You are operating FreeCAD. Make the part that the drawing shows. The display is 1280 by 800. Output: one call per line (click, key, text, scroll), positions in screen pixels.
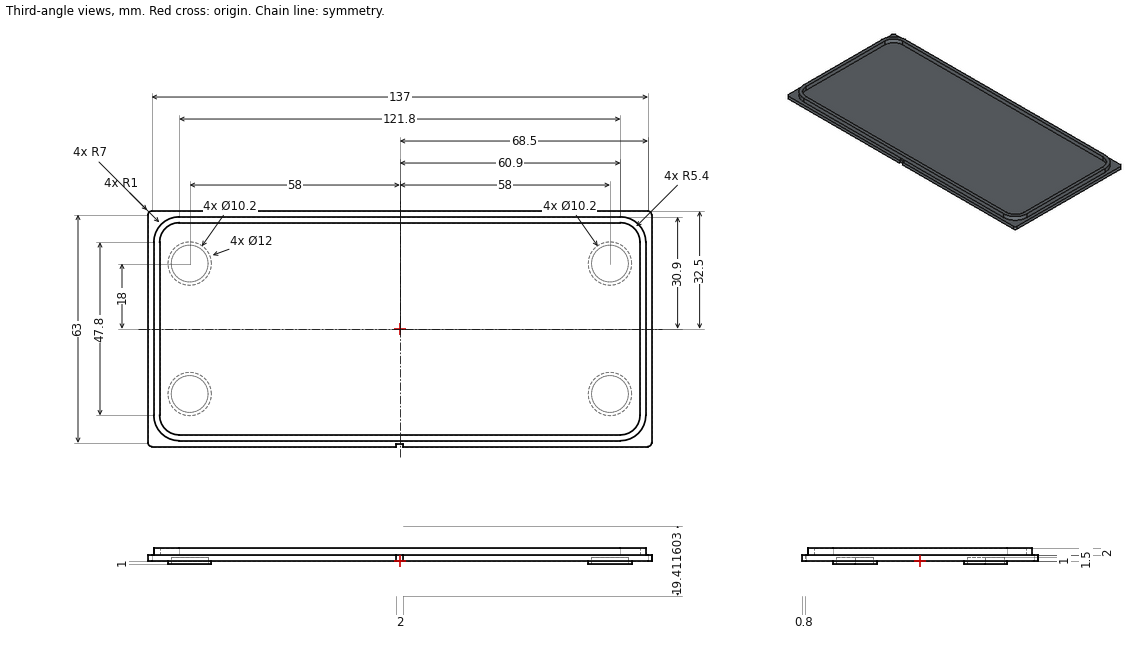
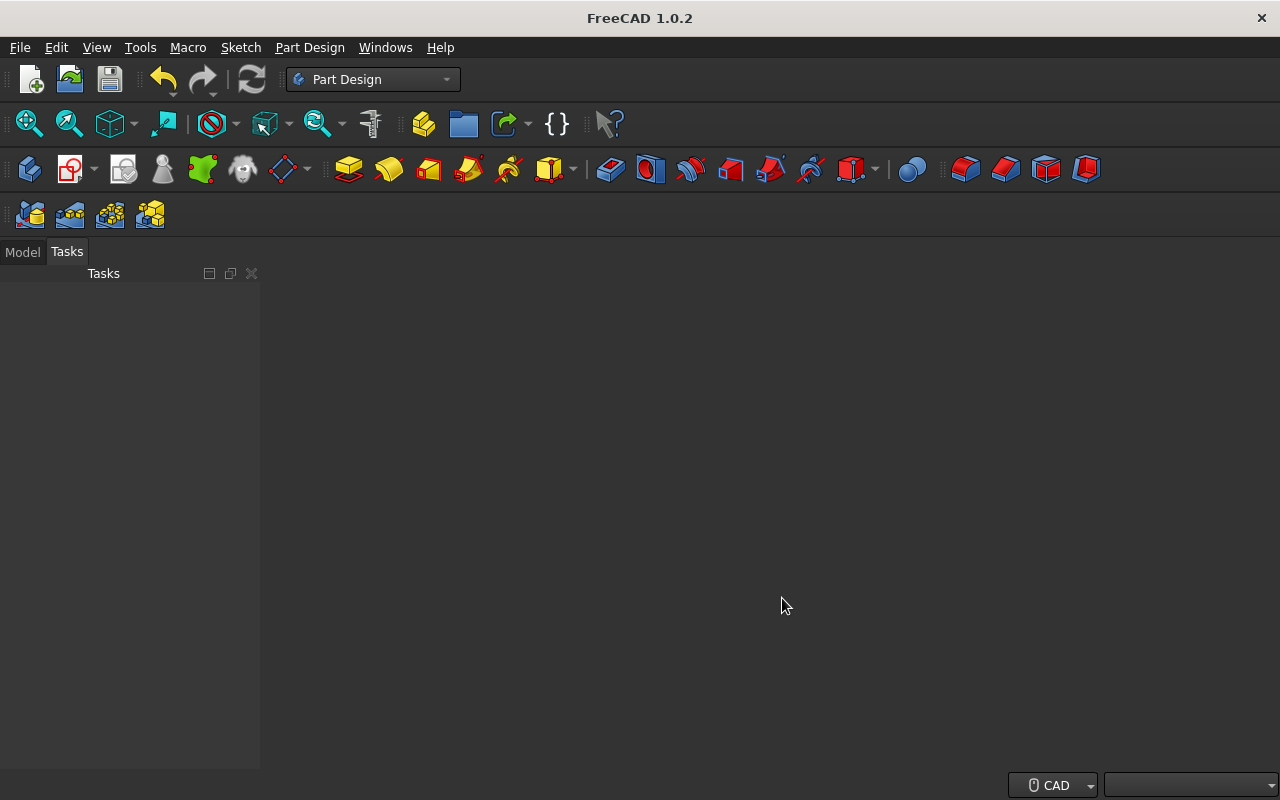
click(30, 80)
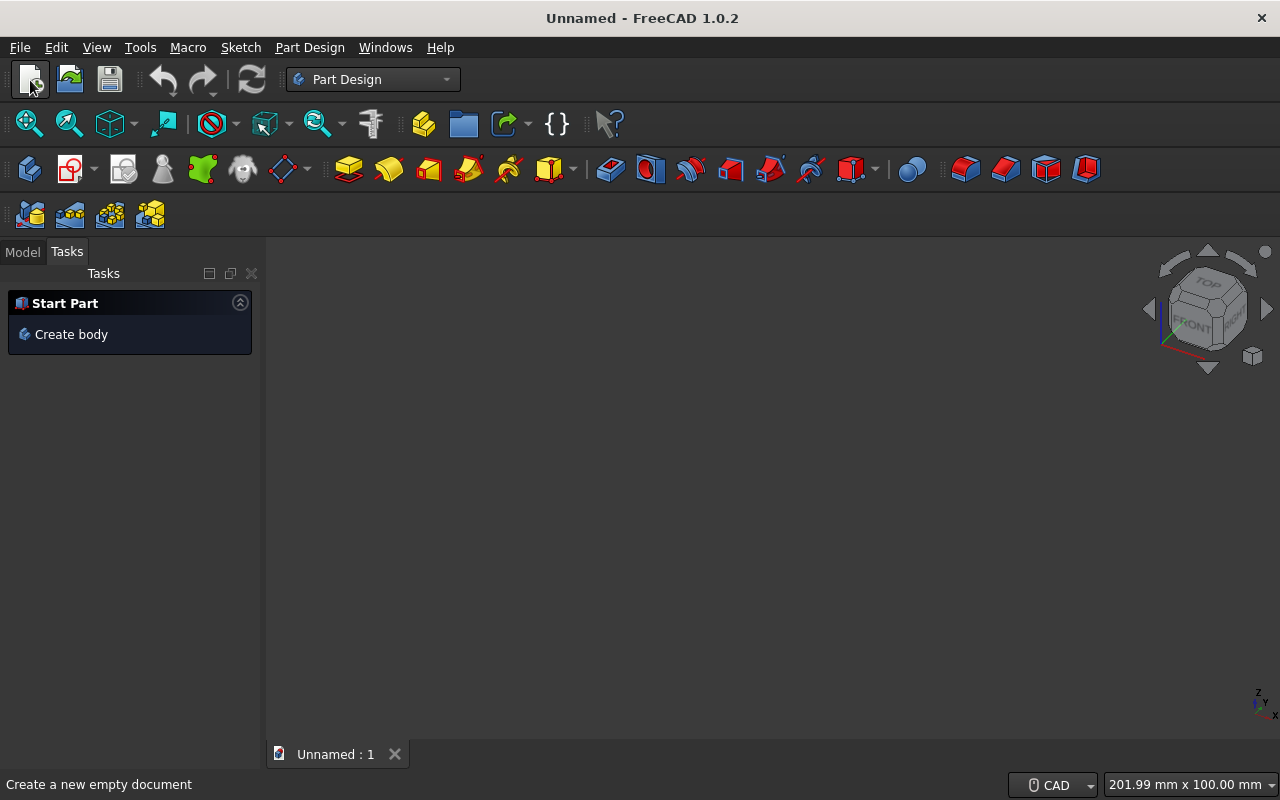
click(70, 170)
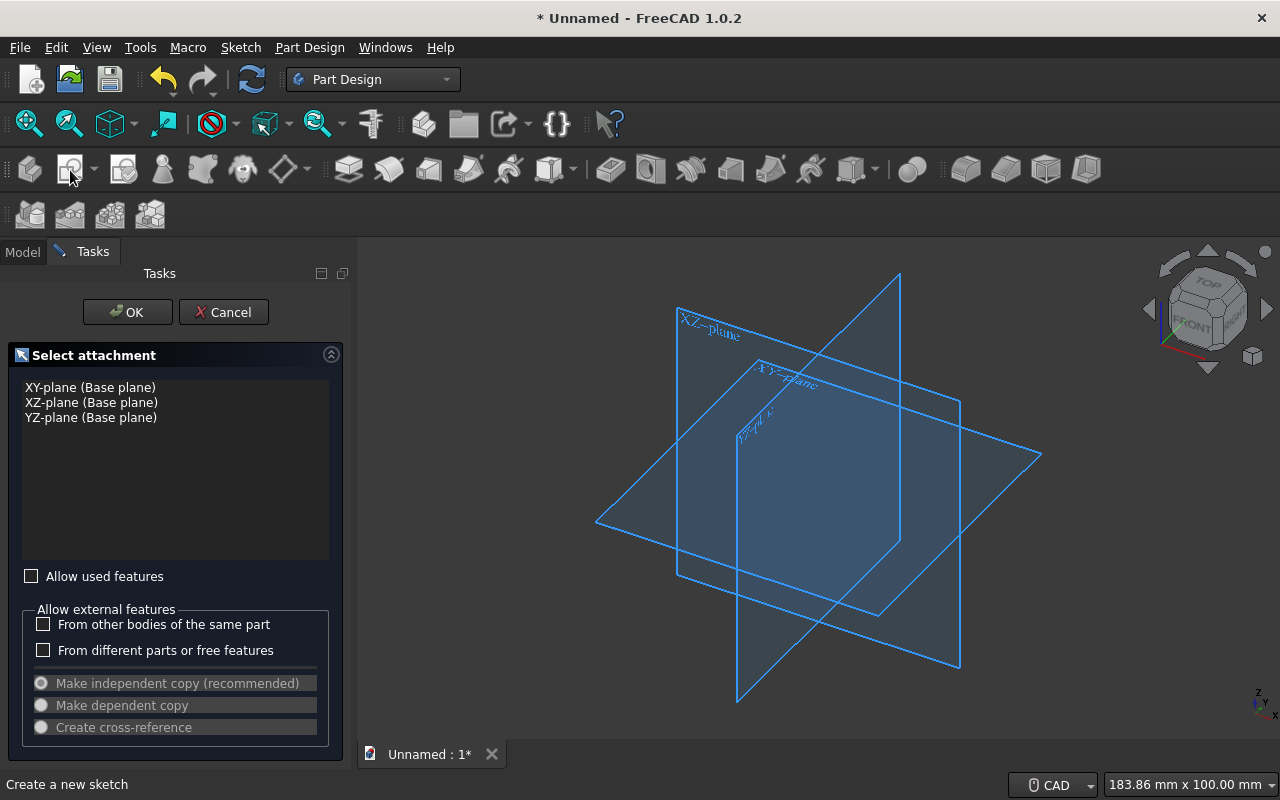
click(82, 388)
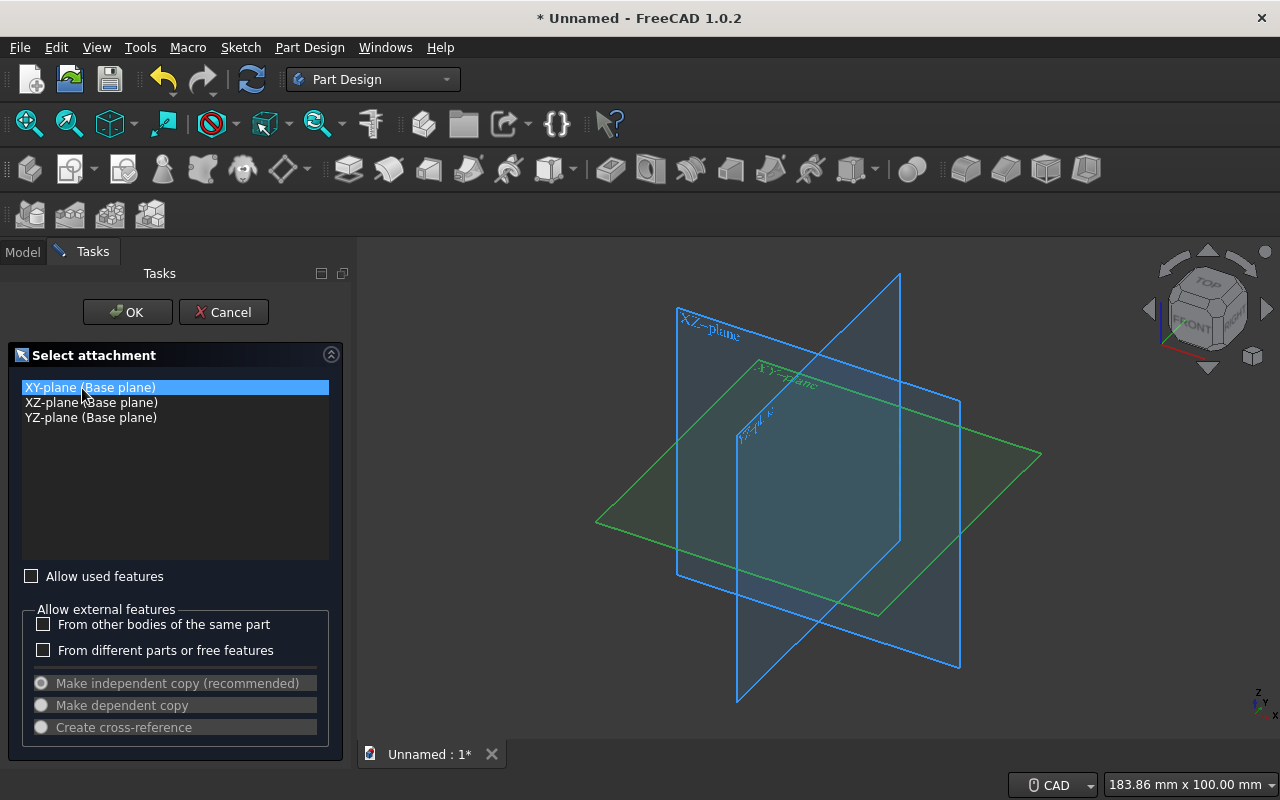
click(128, 312)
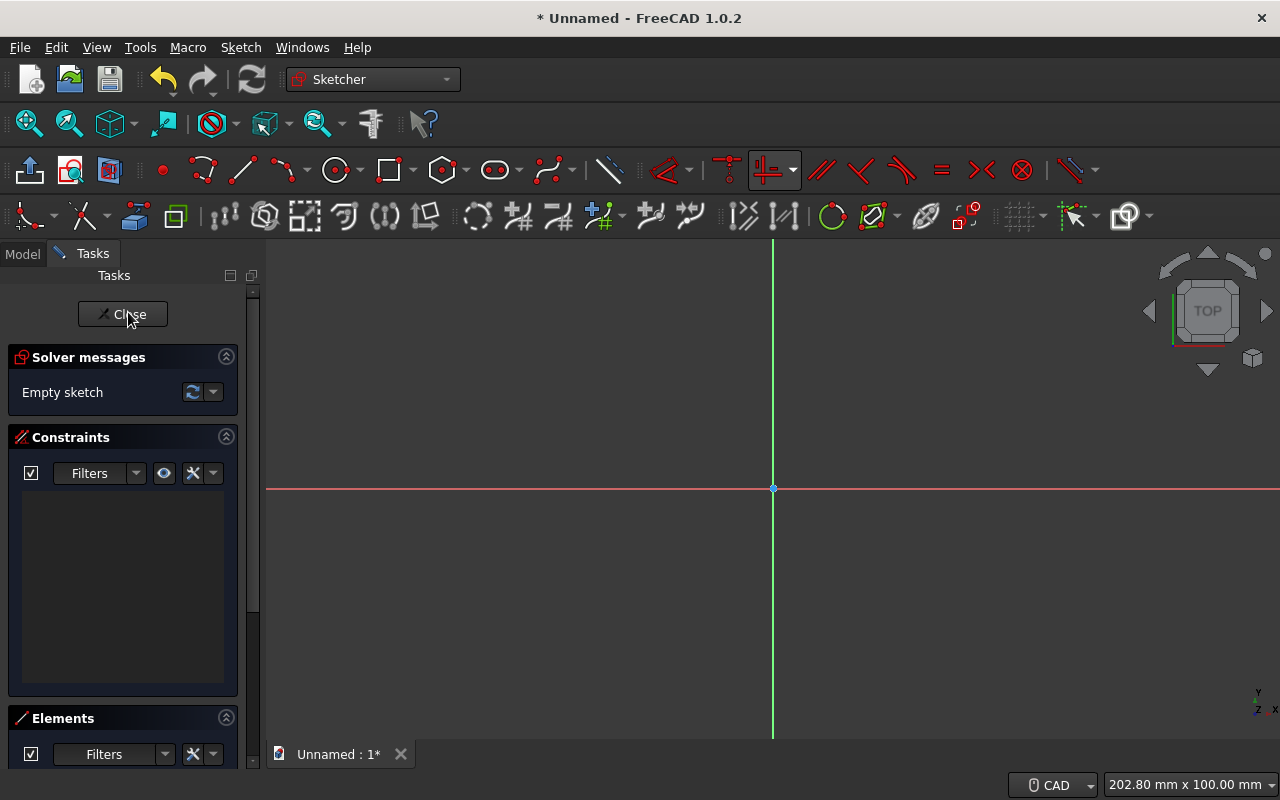
scroll(395, 489, down, 1)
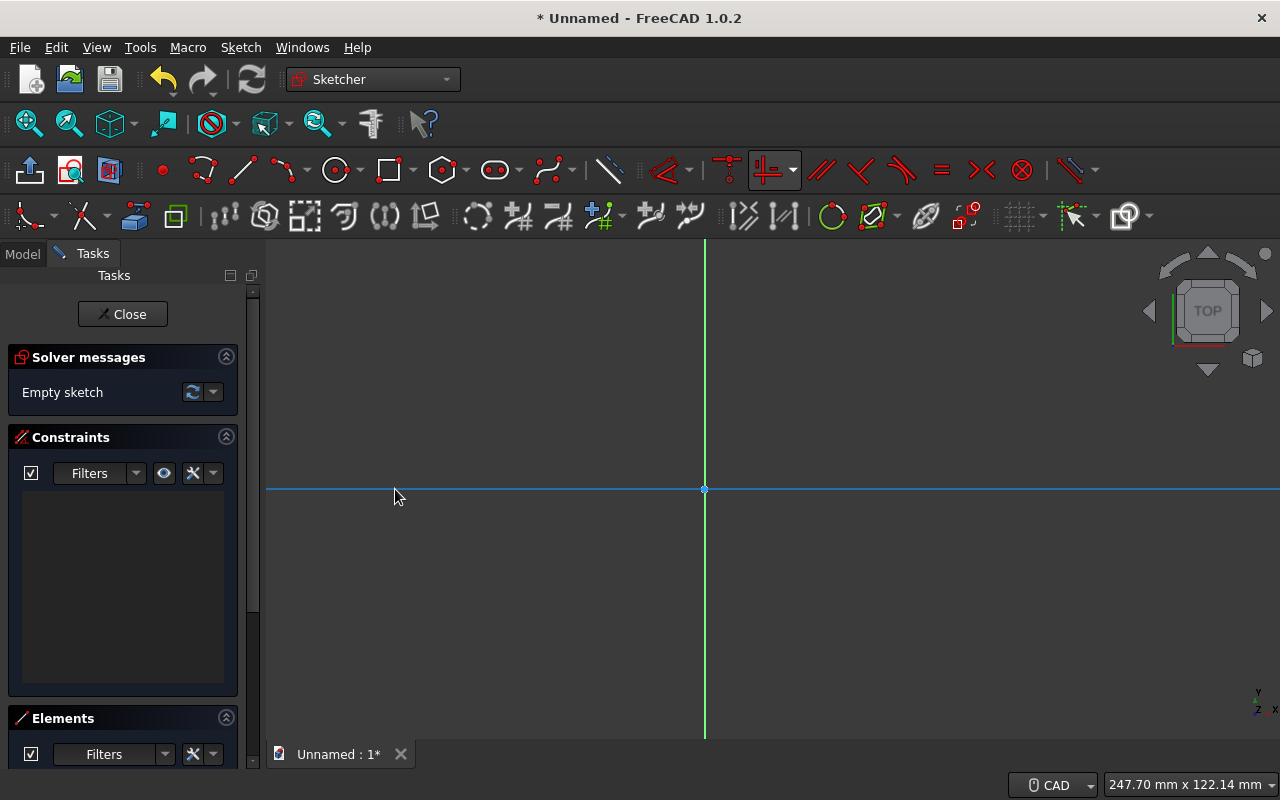
click(244, 170)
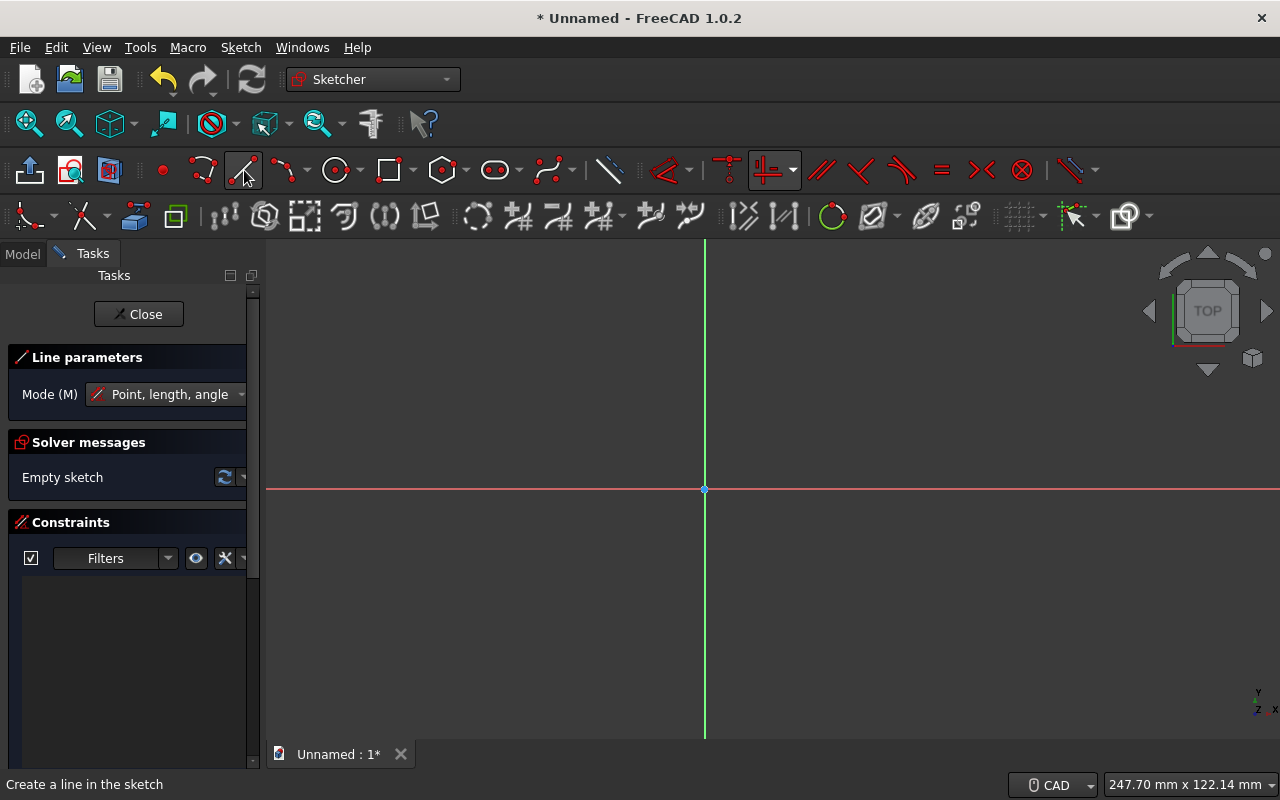
click(985, 356)
click(424, 356)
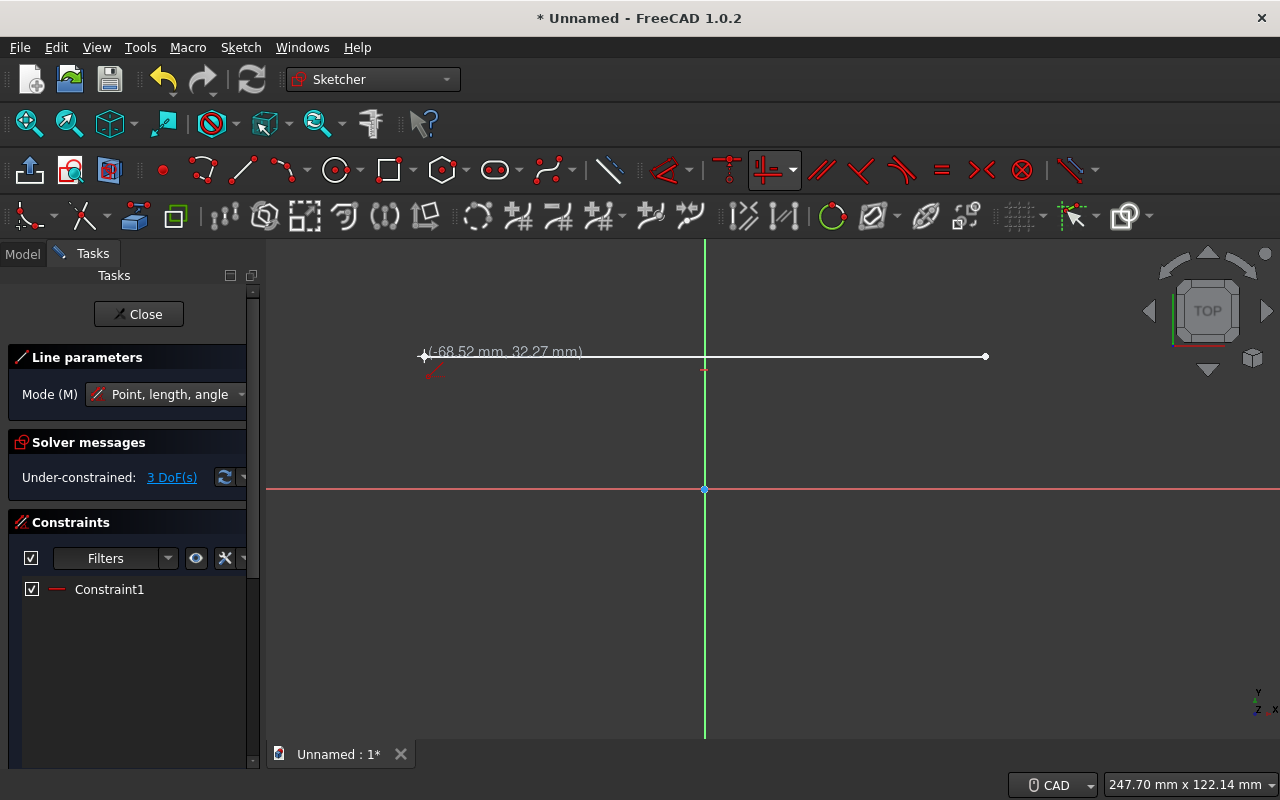
scroll(420, 360, up, 6)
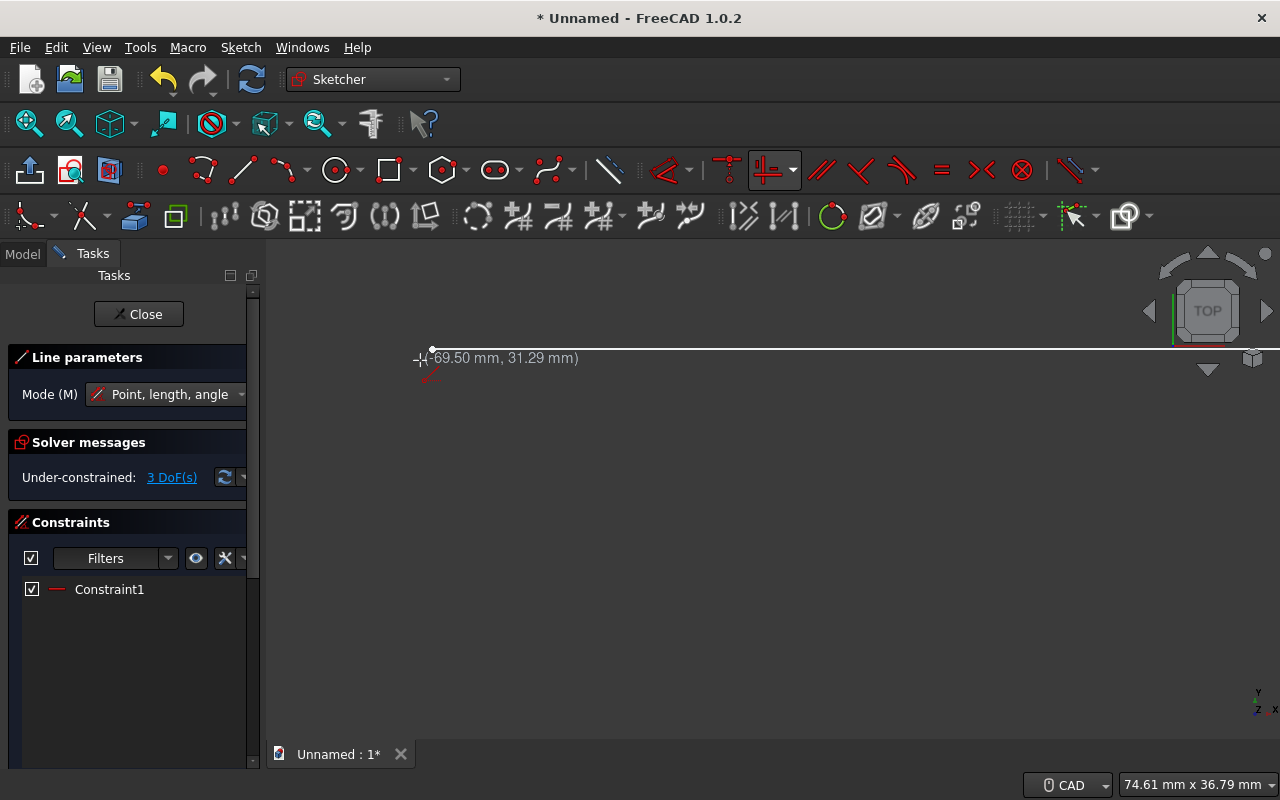
click(420, 360)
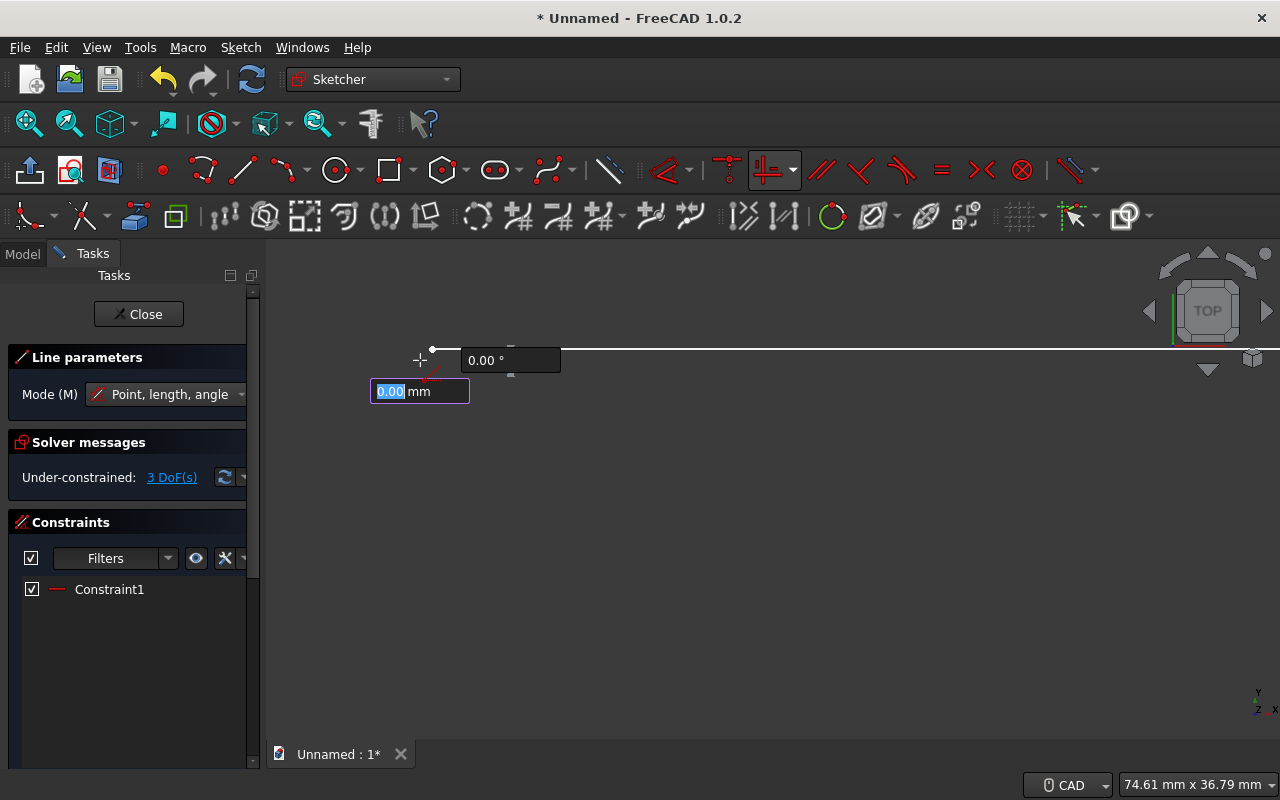
scroll(420, 360, down, 6)